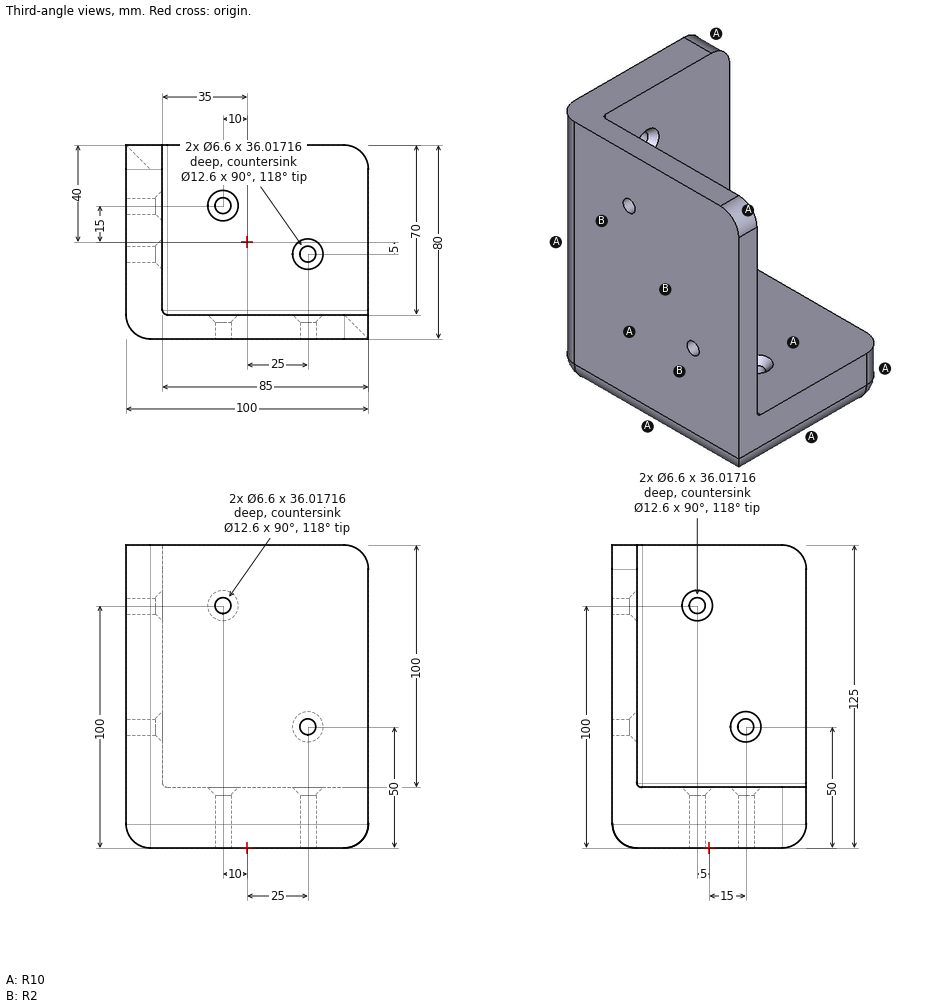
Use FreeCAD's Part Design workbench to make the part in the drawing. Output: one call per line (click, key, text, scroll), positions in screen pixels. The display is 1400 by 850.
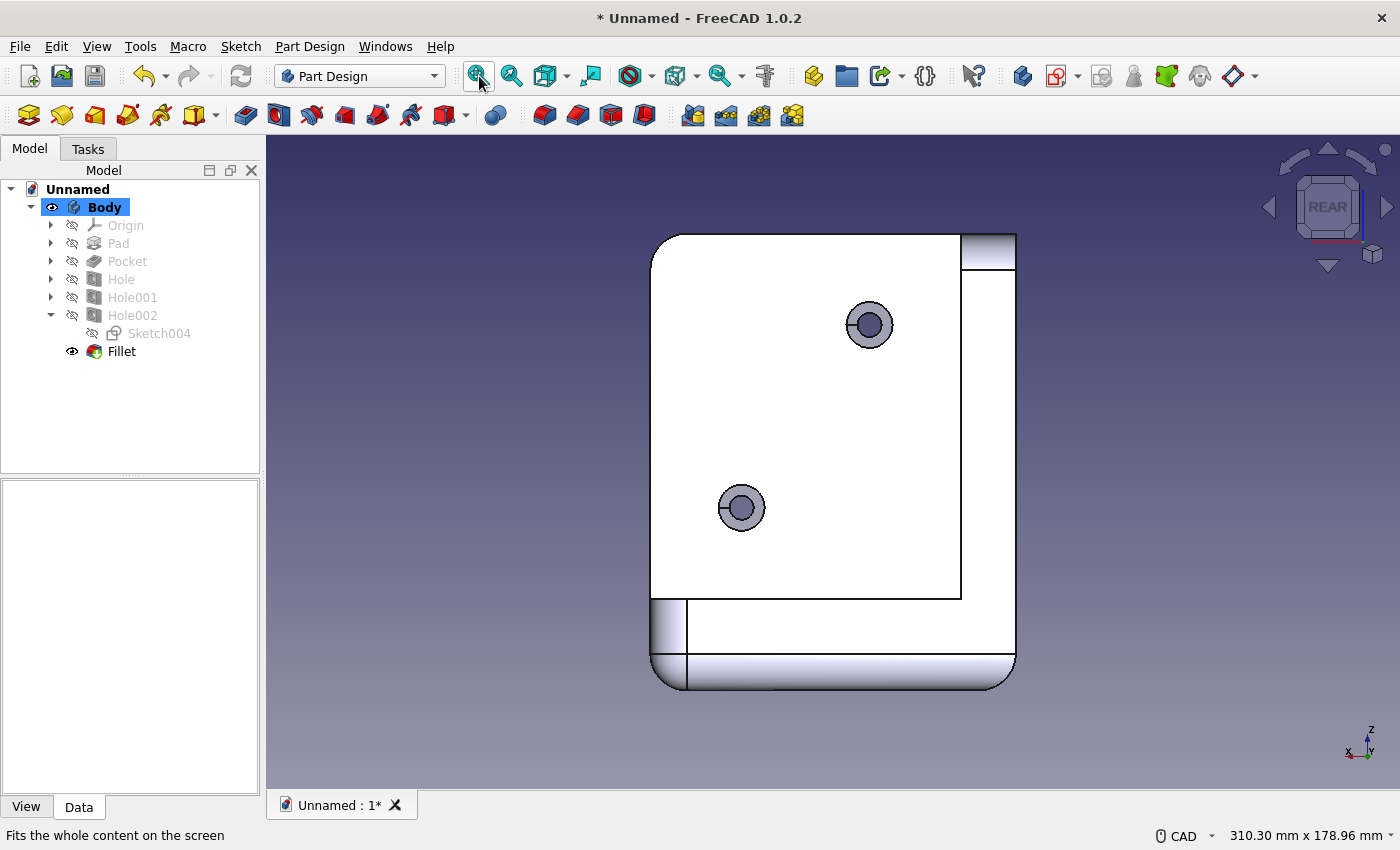
key(6)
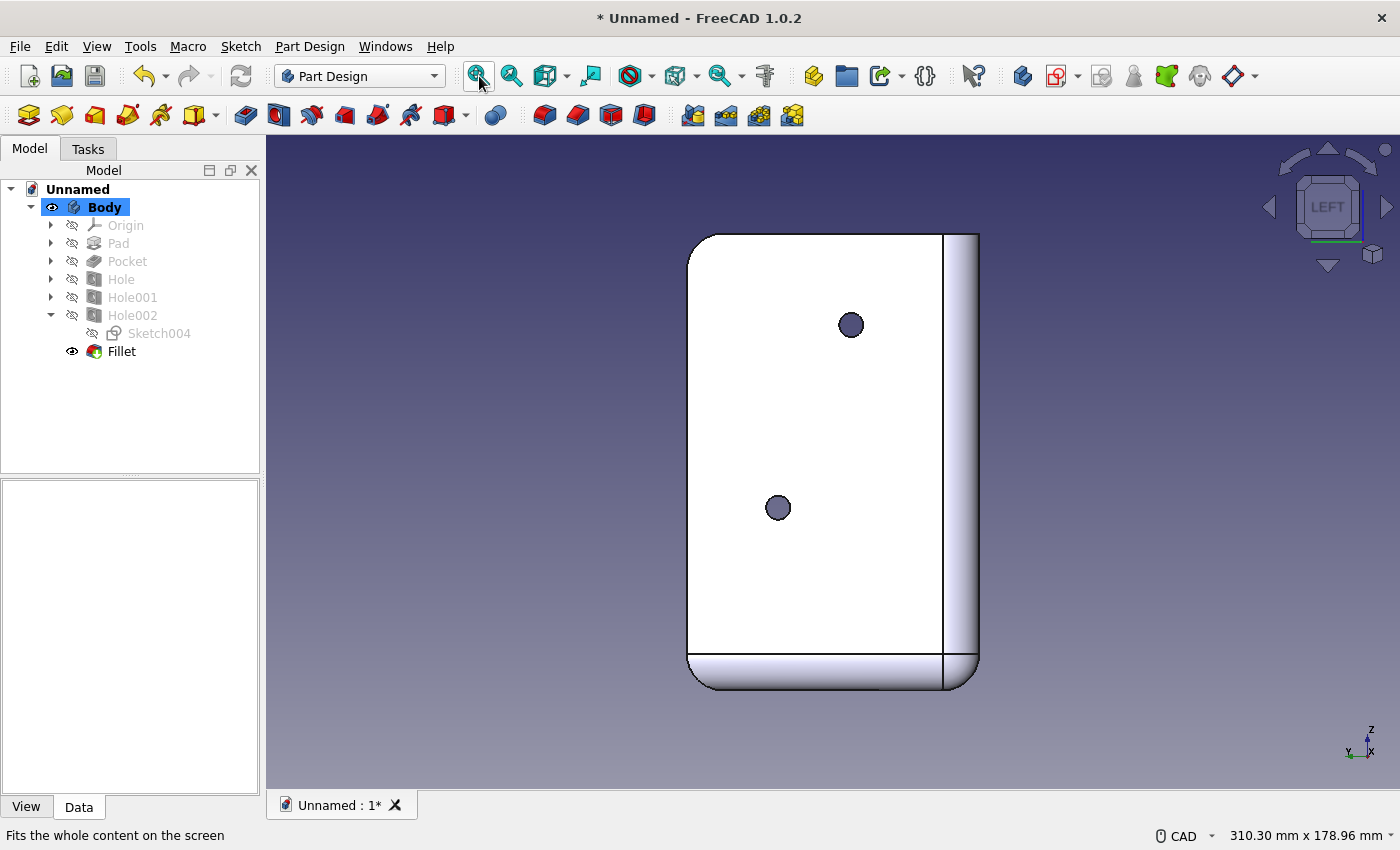
key(v)
key(3)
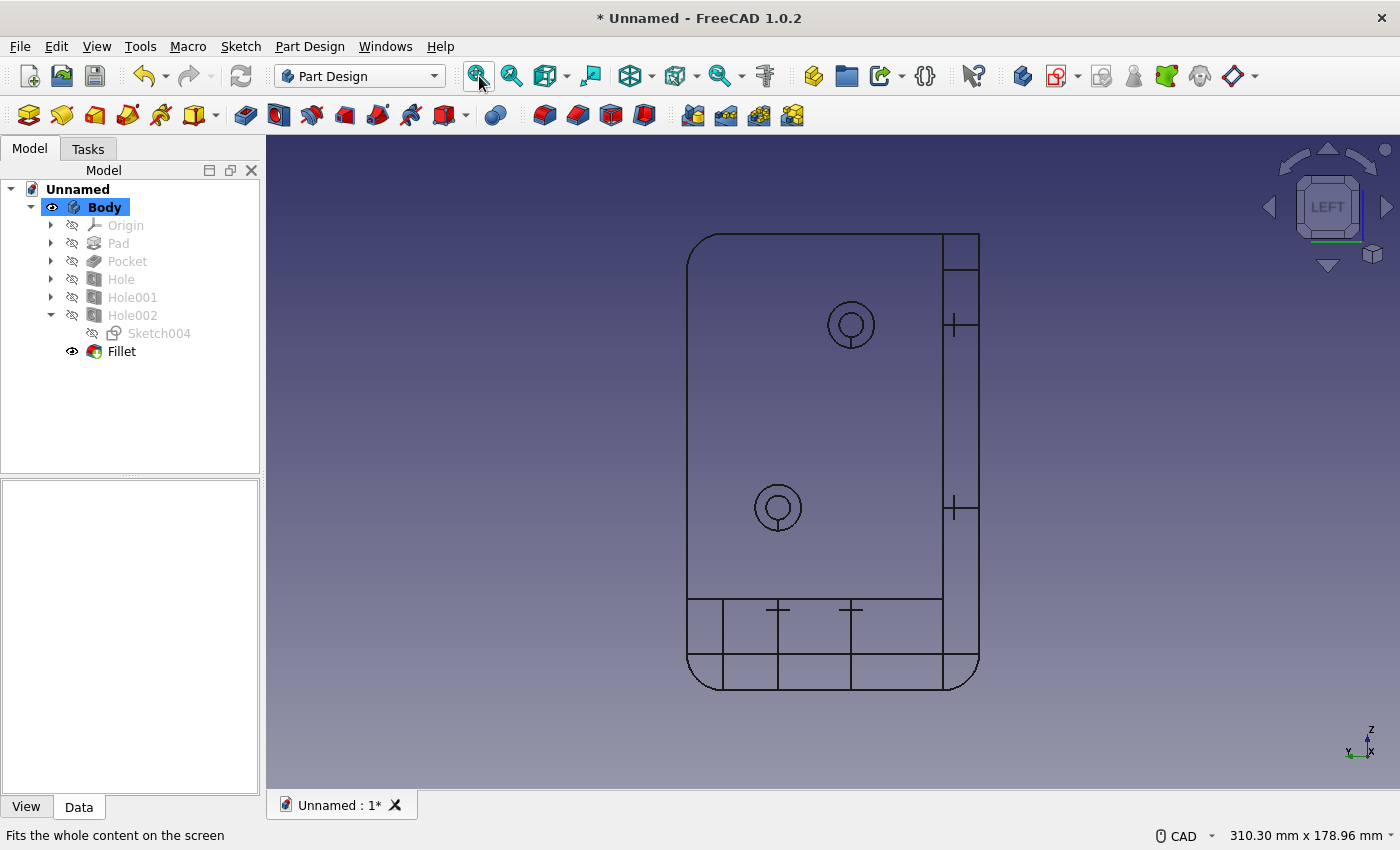
key(0)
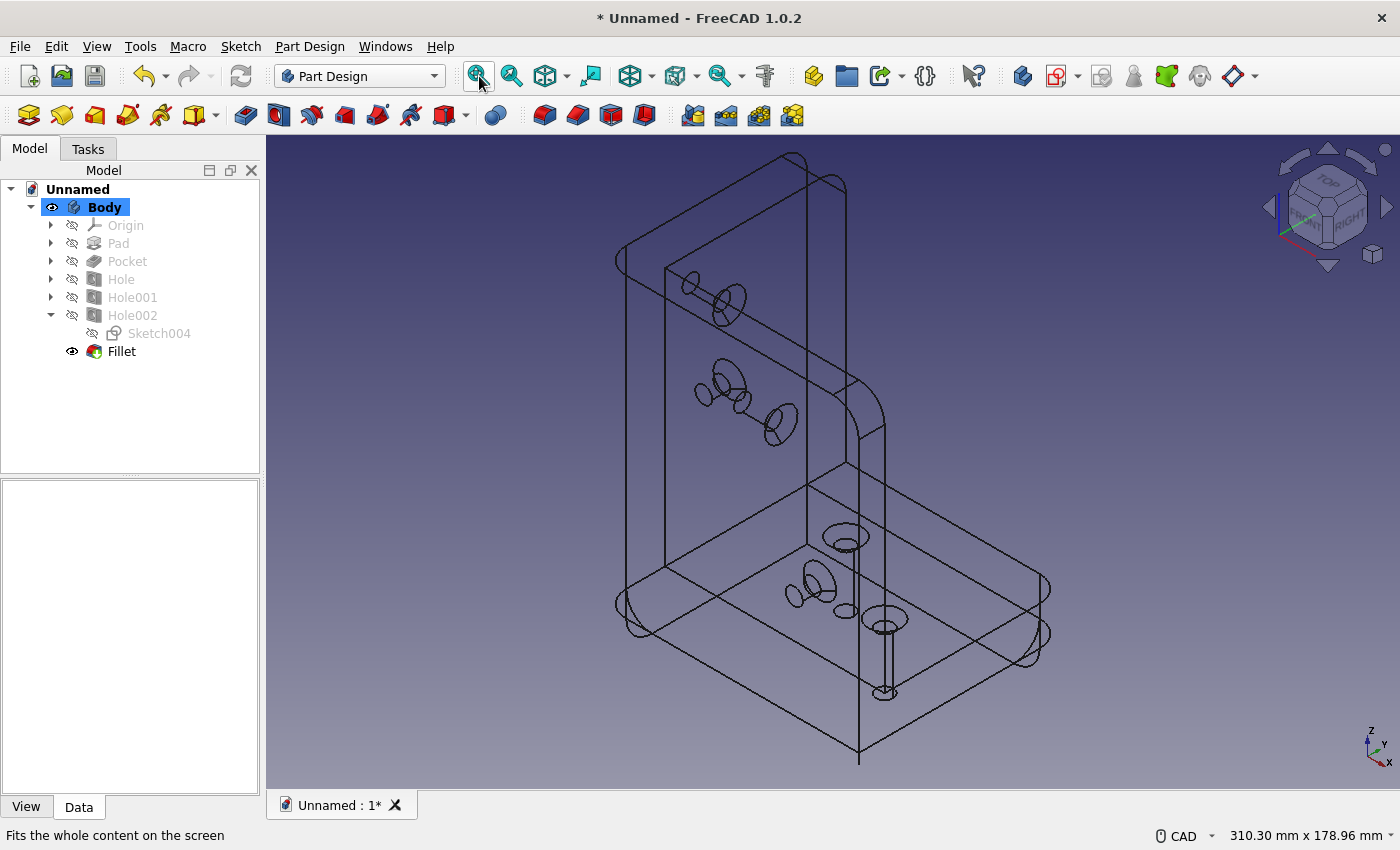
click(755, 513)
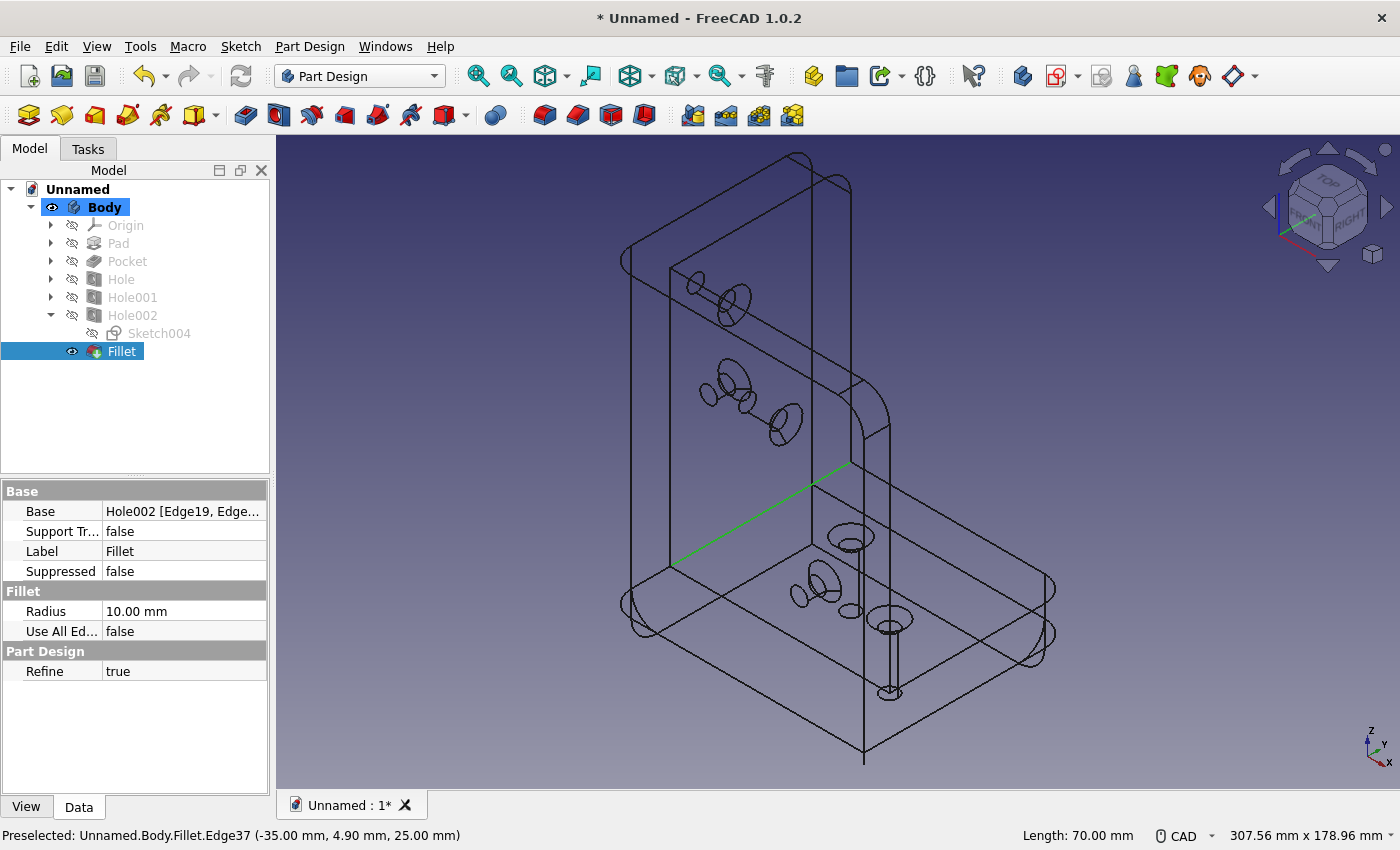
click(670, 416, ctrl)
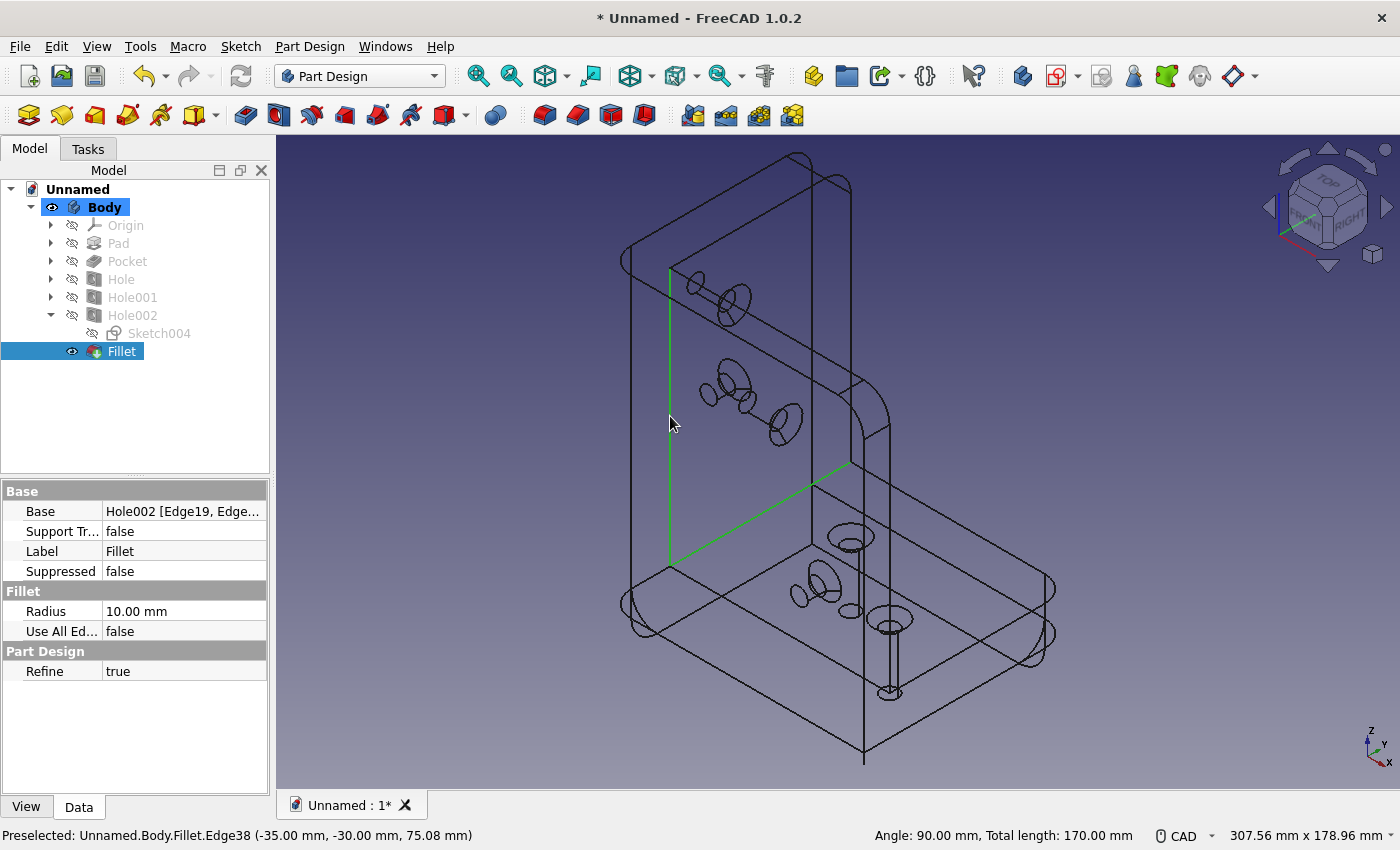
click(780, 629, ctrl)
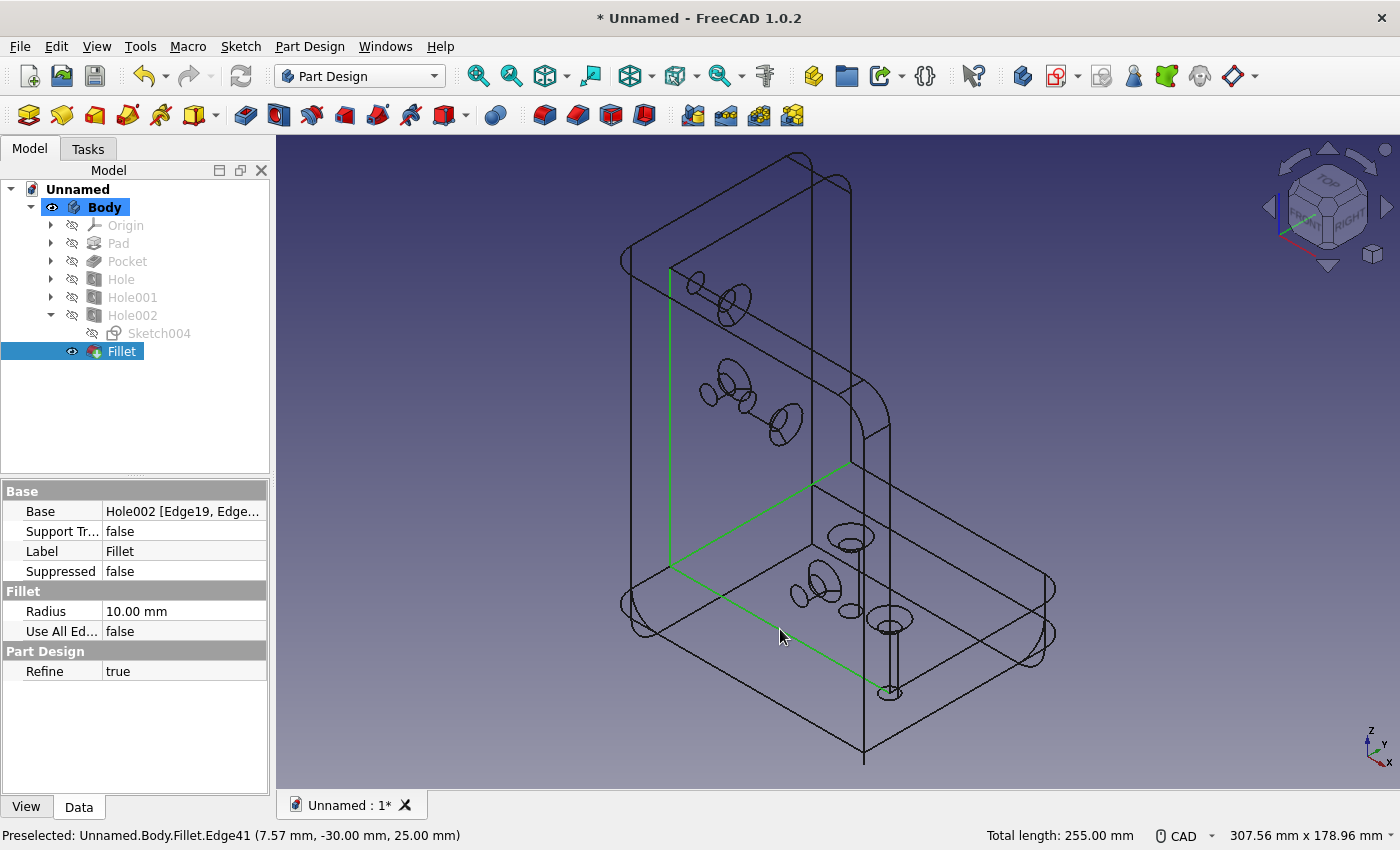
key(v)
key(1)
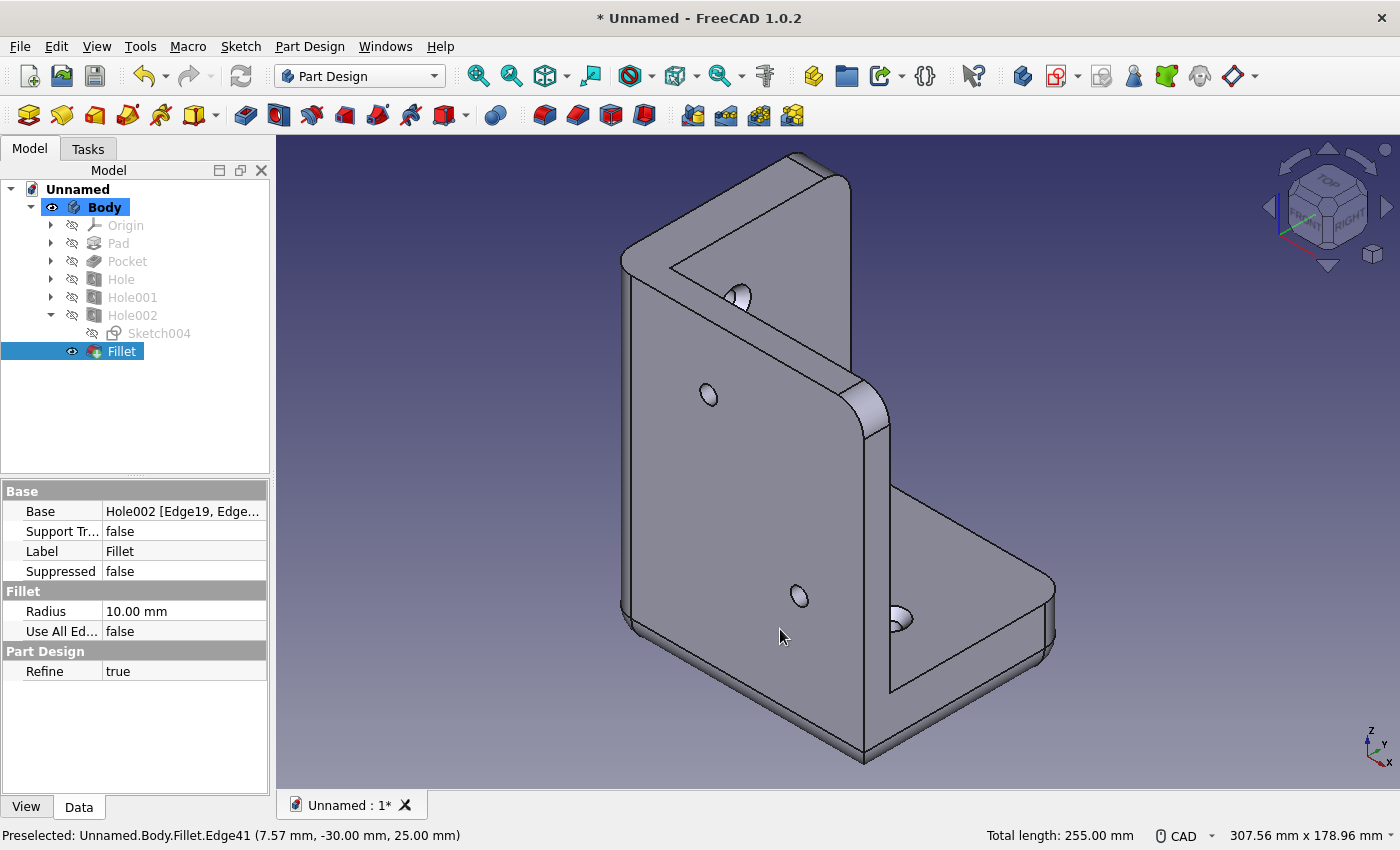
click(545, 116)